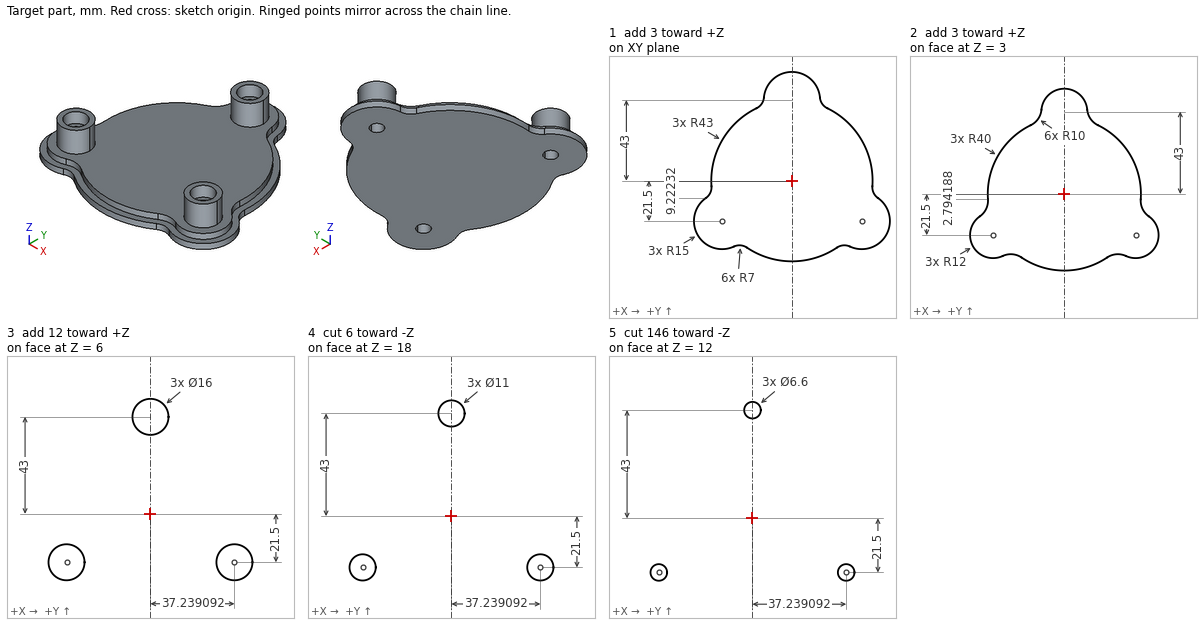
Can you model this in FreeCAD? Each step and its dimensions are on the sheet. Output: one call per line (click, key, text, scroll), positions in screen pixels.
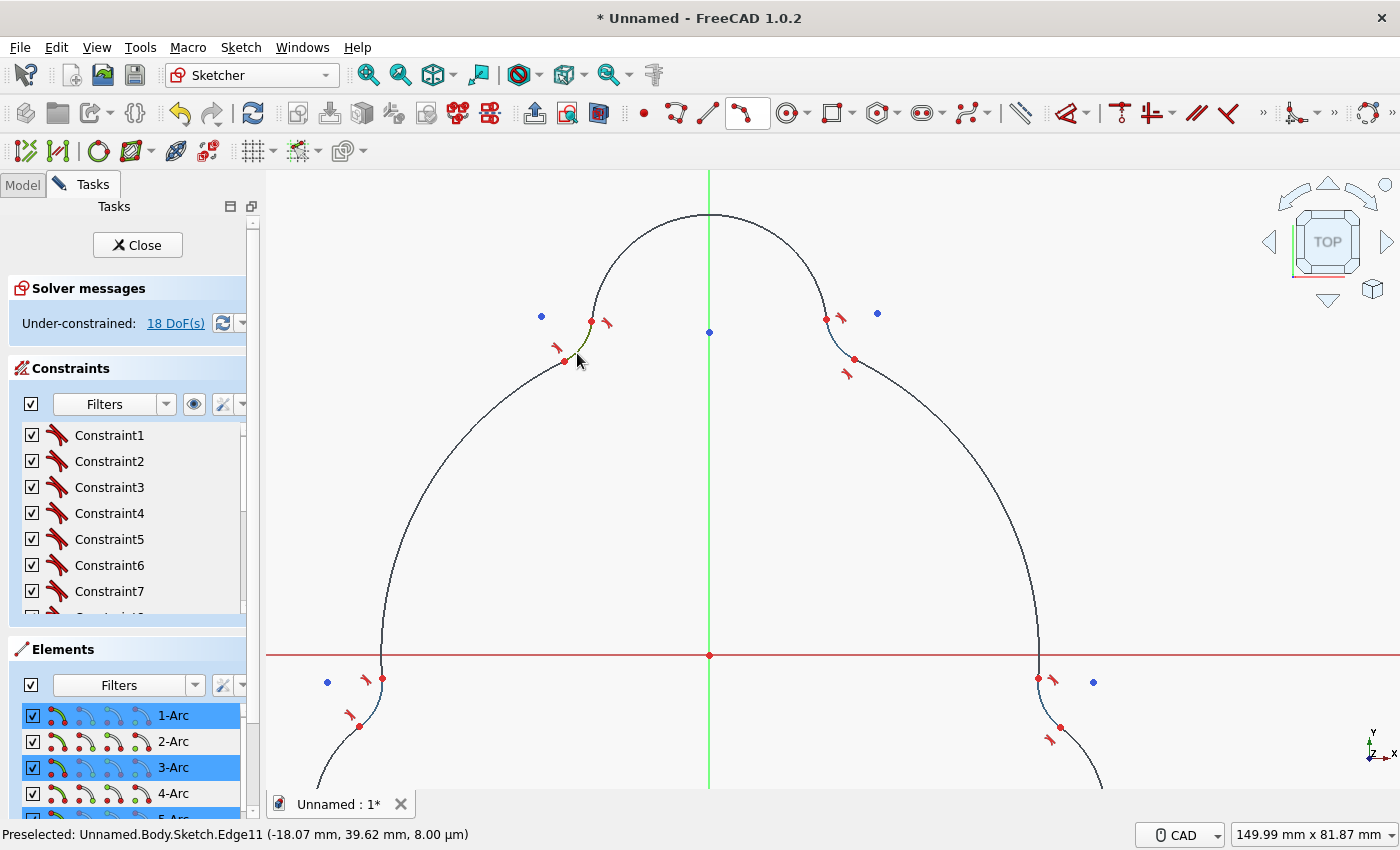
key(e)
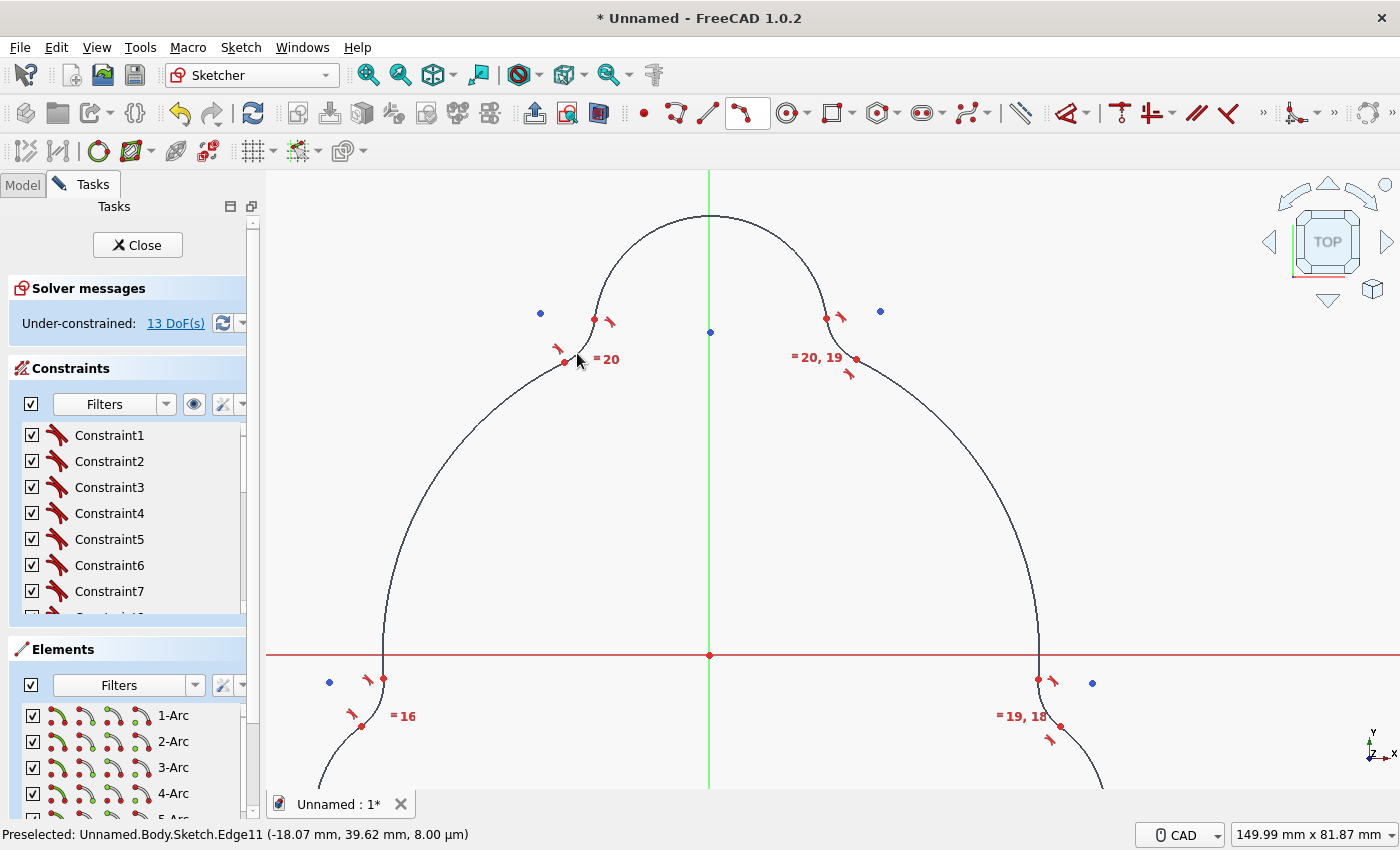
scroll(832, 335, down, 3)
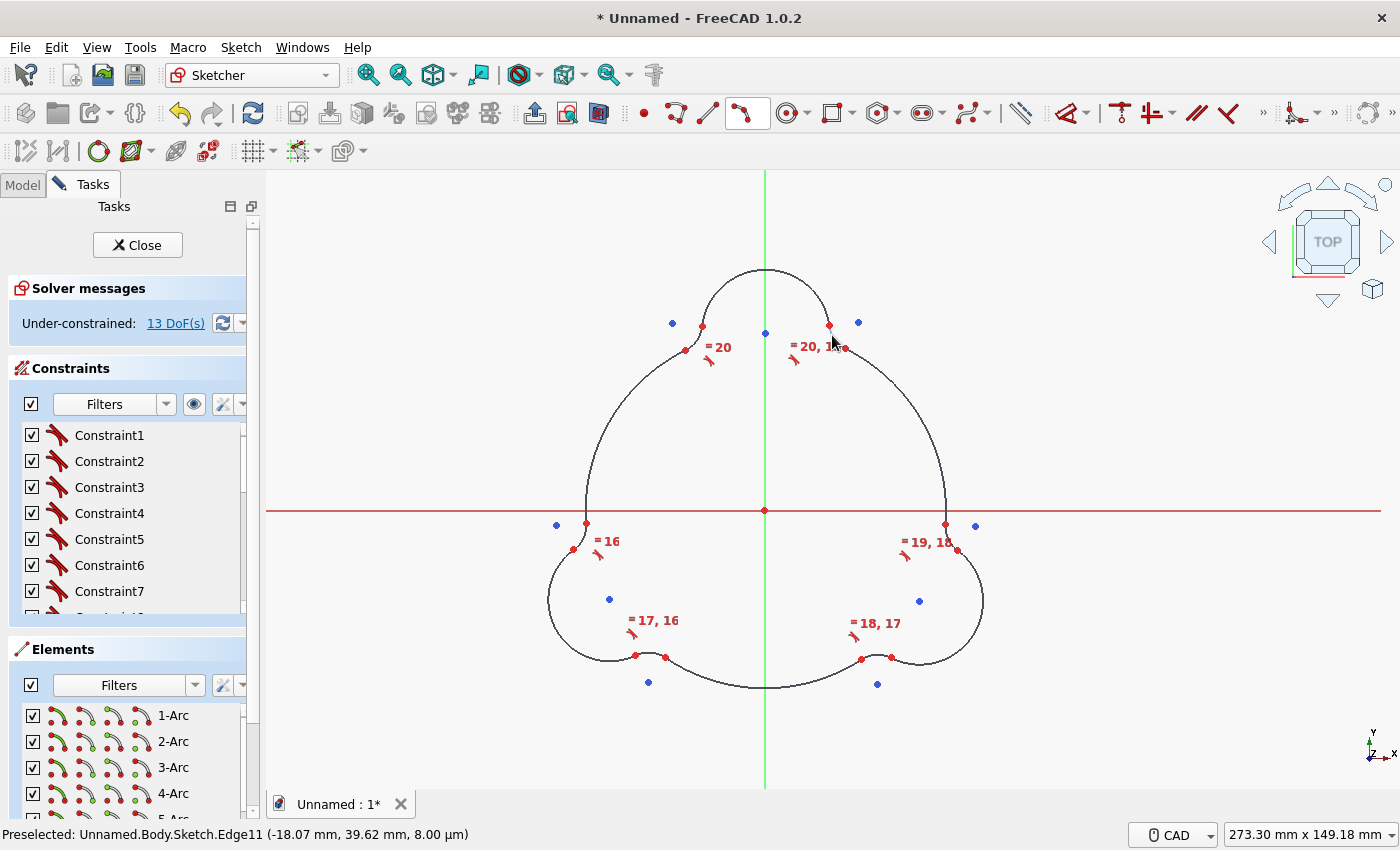
click(548, 596)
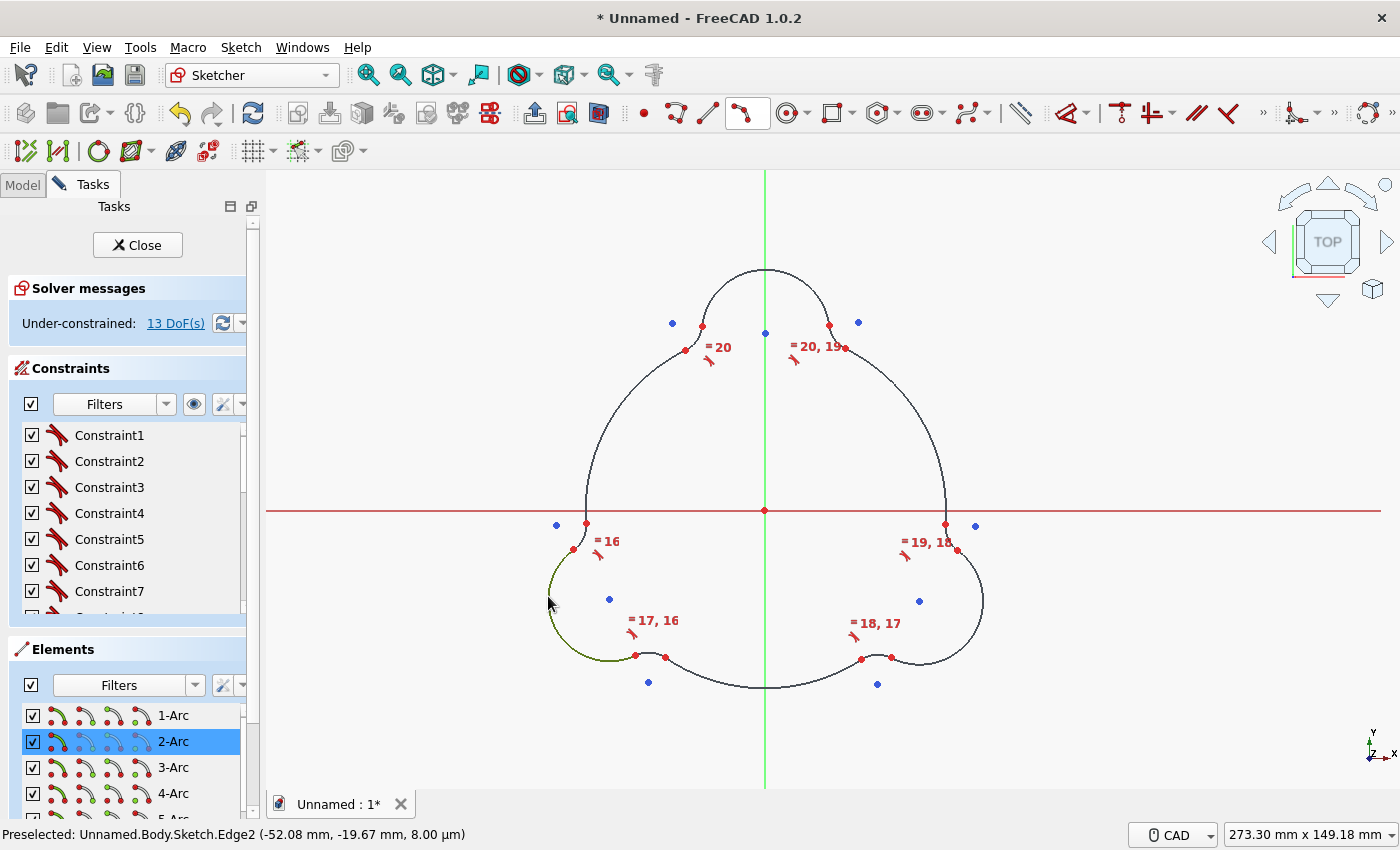
click(946, 659)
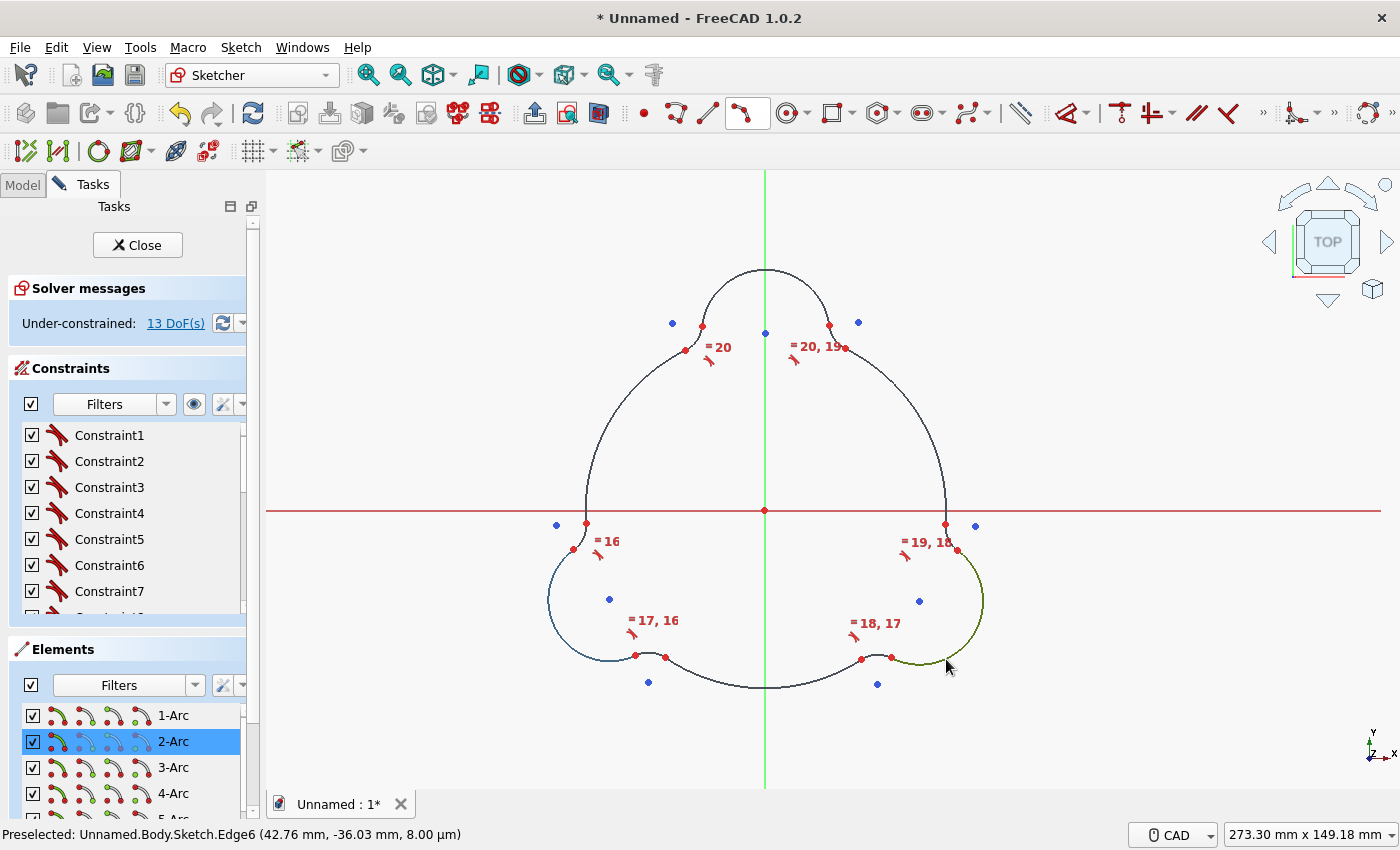
click(800, 280)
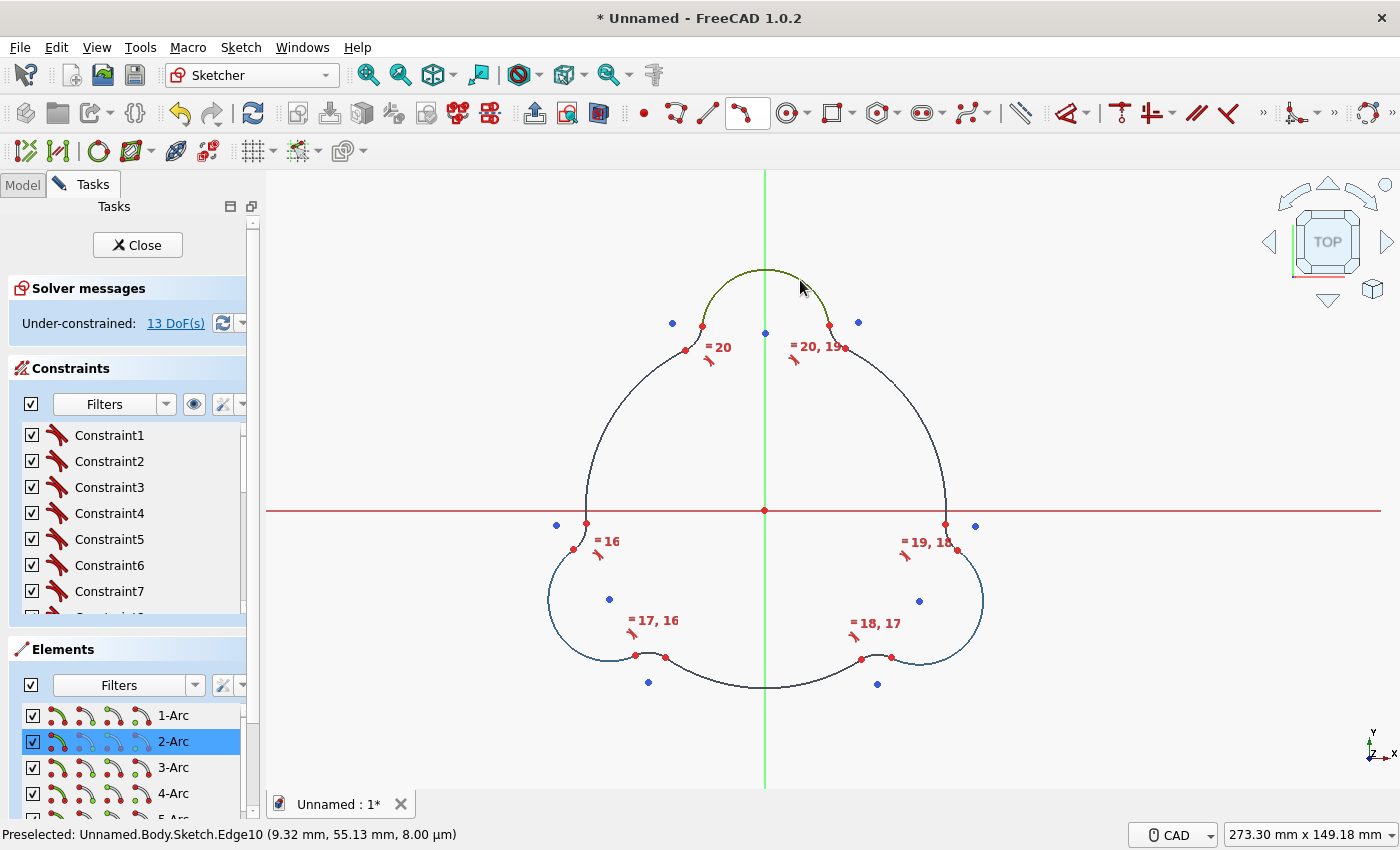
key(e)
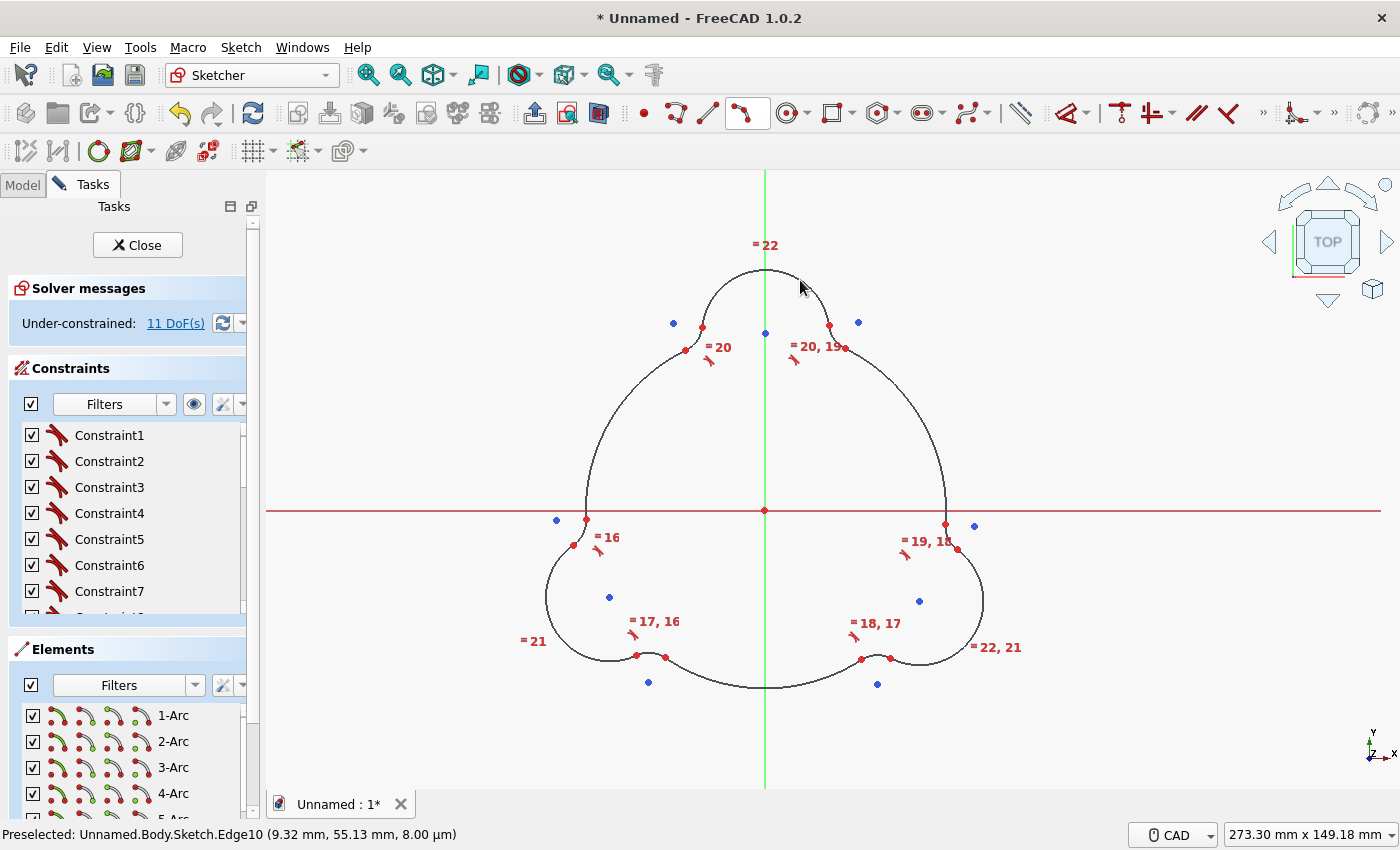
click(722, 683)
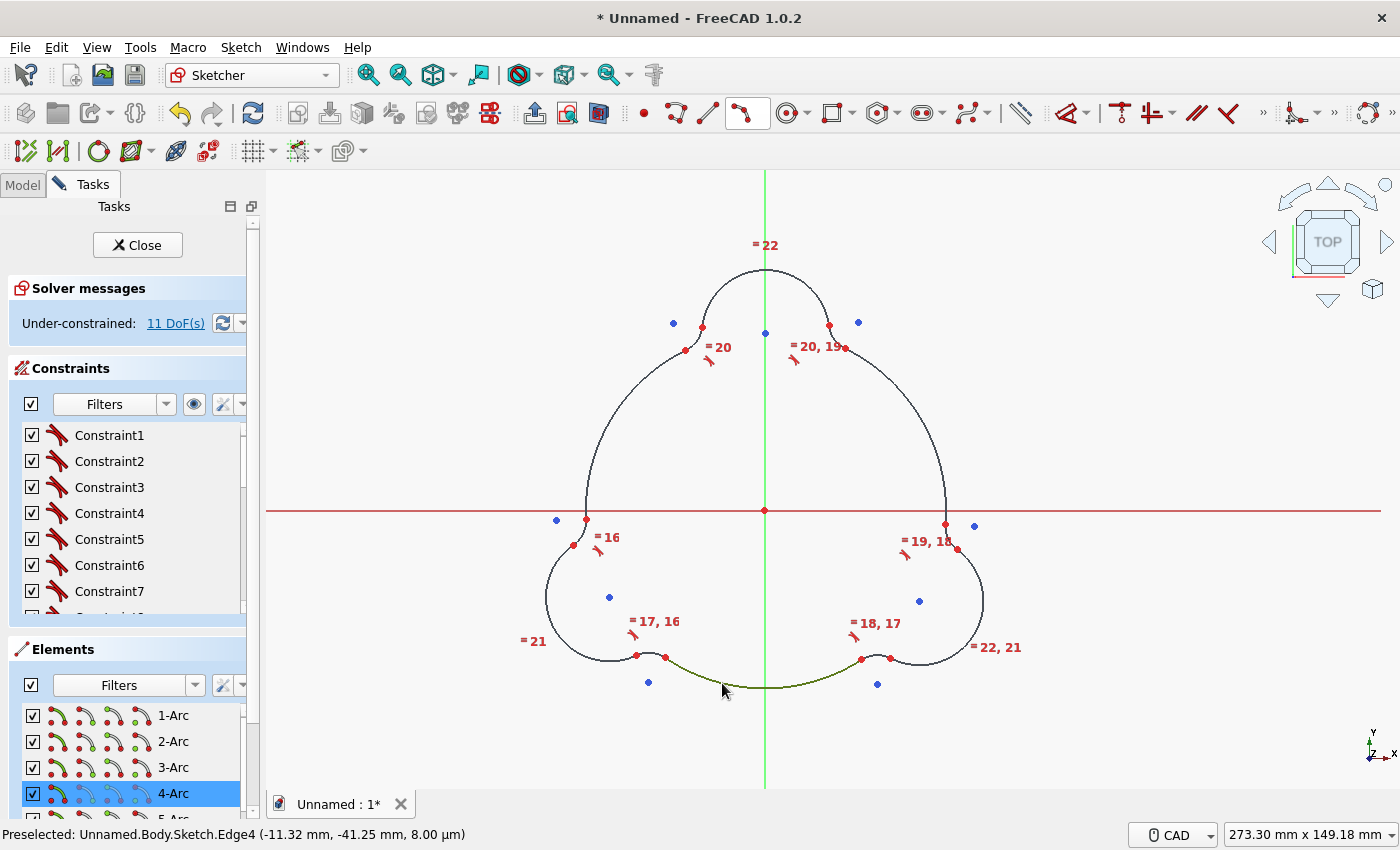
click(939, 460)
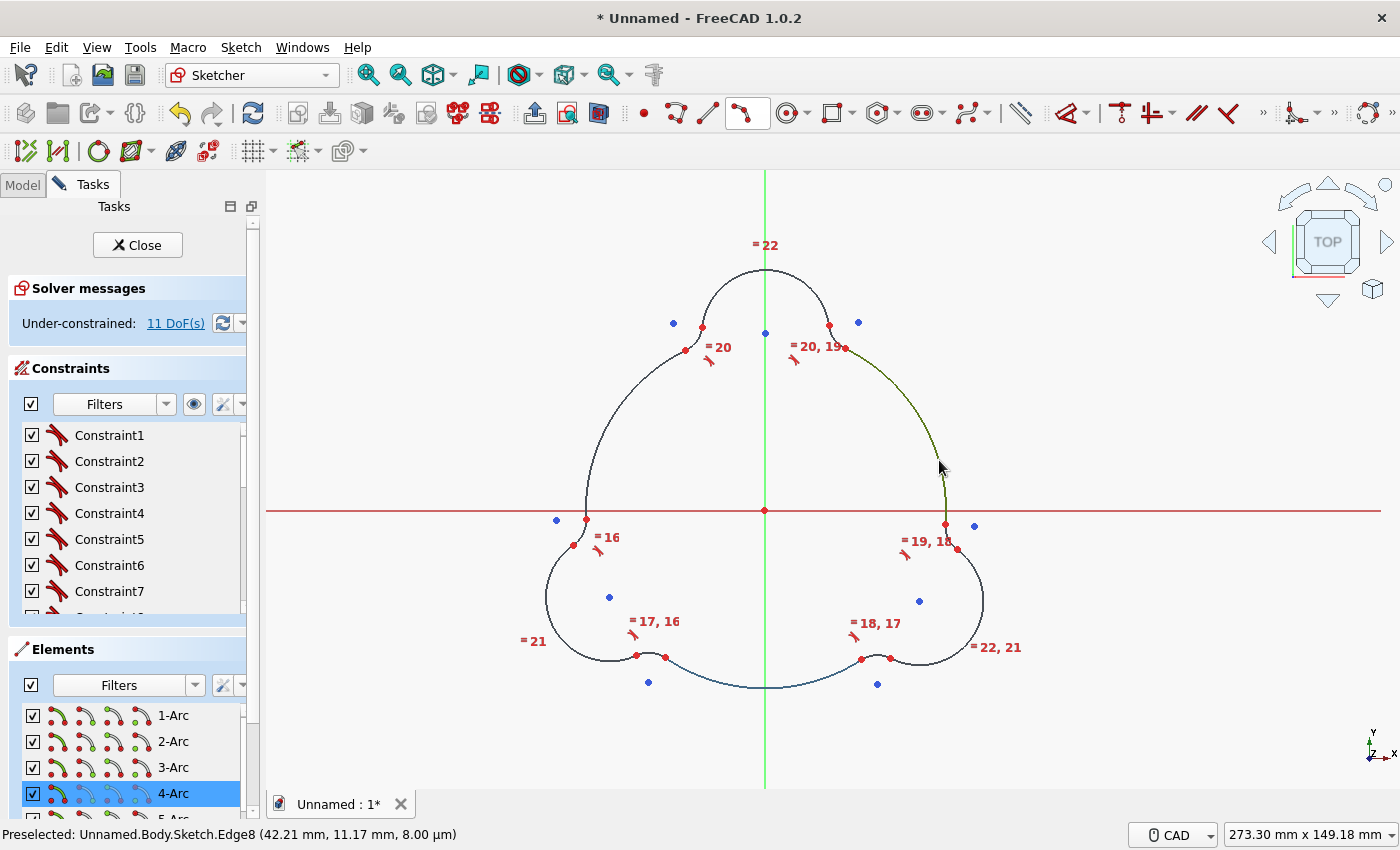
click(636, 387)